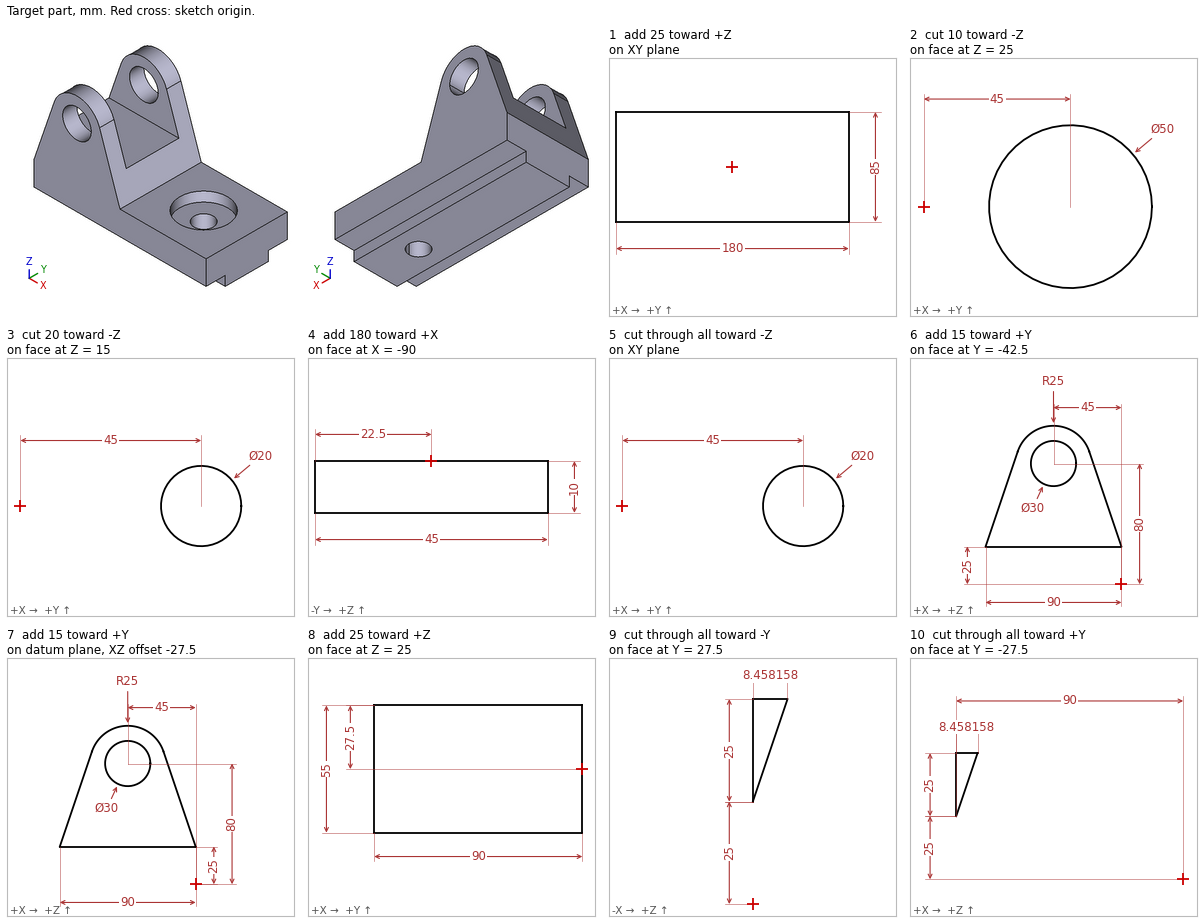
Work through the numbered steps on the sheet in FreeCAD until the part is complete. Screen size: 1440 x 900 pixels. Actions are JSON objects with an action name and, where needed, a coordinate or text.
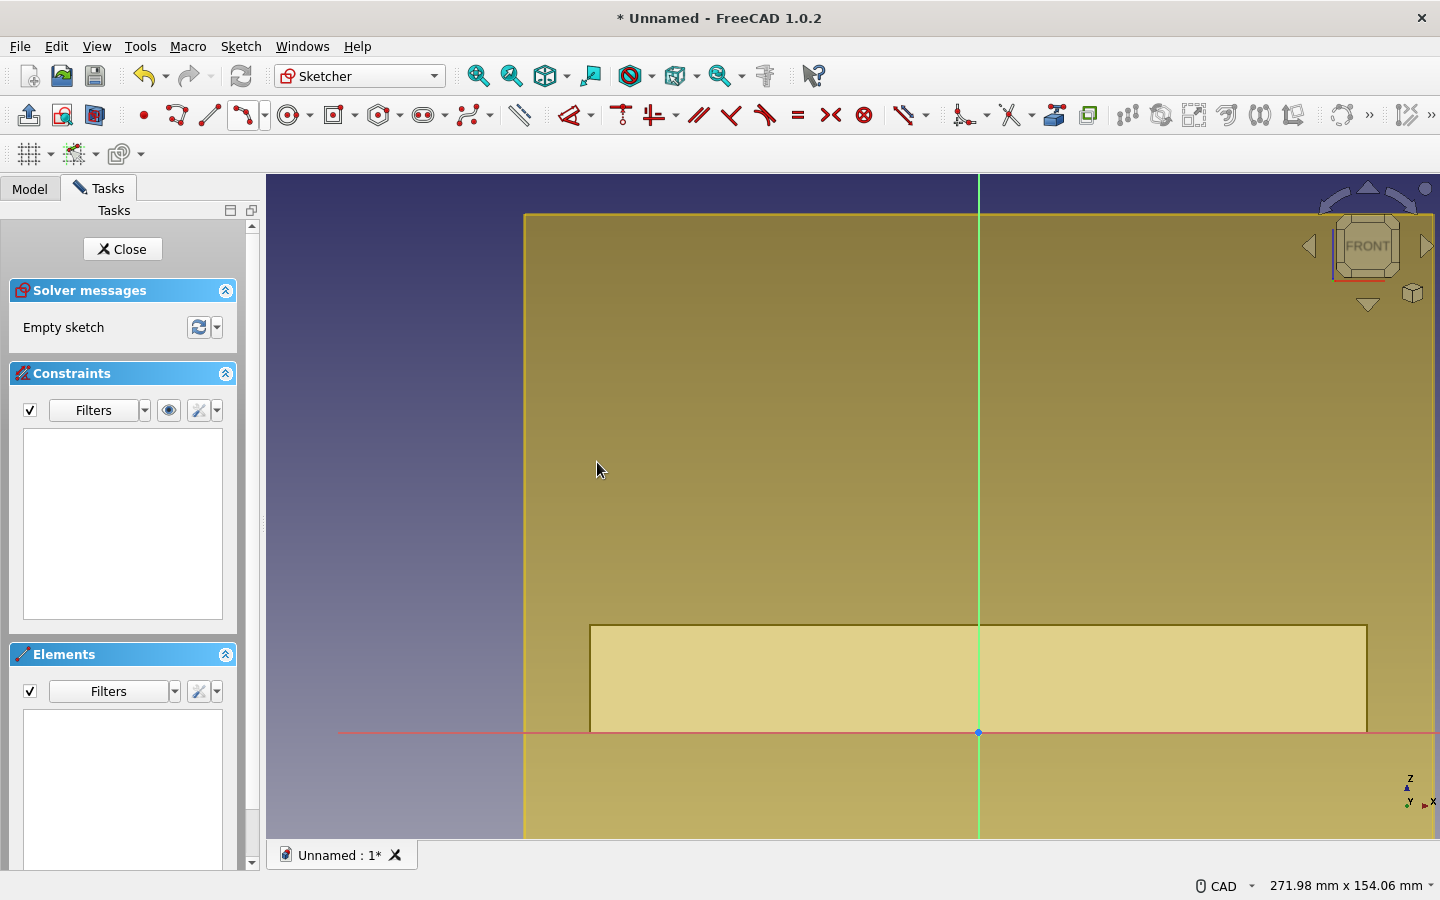
{"action": "left_click", "coordinate": [177, 116]}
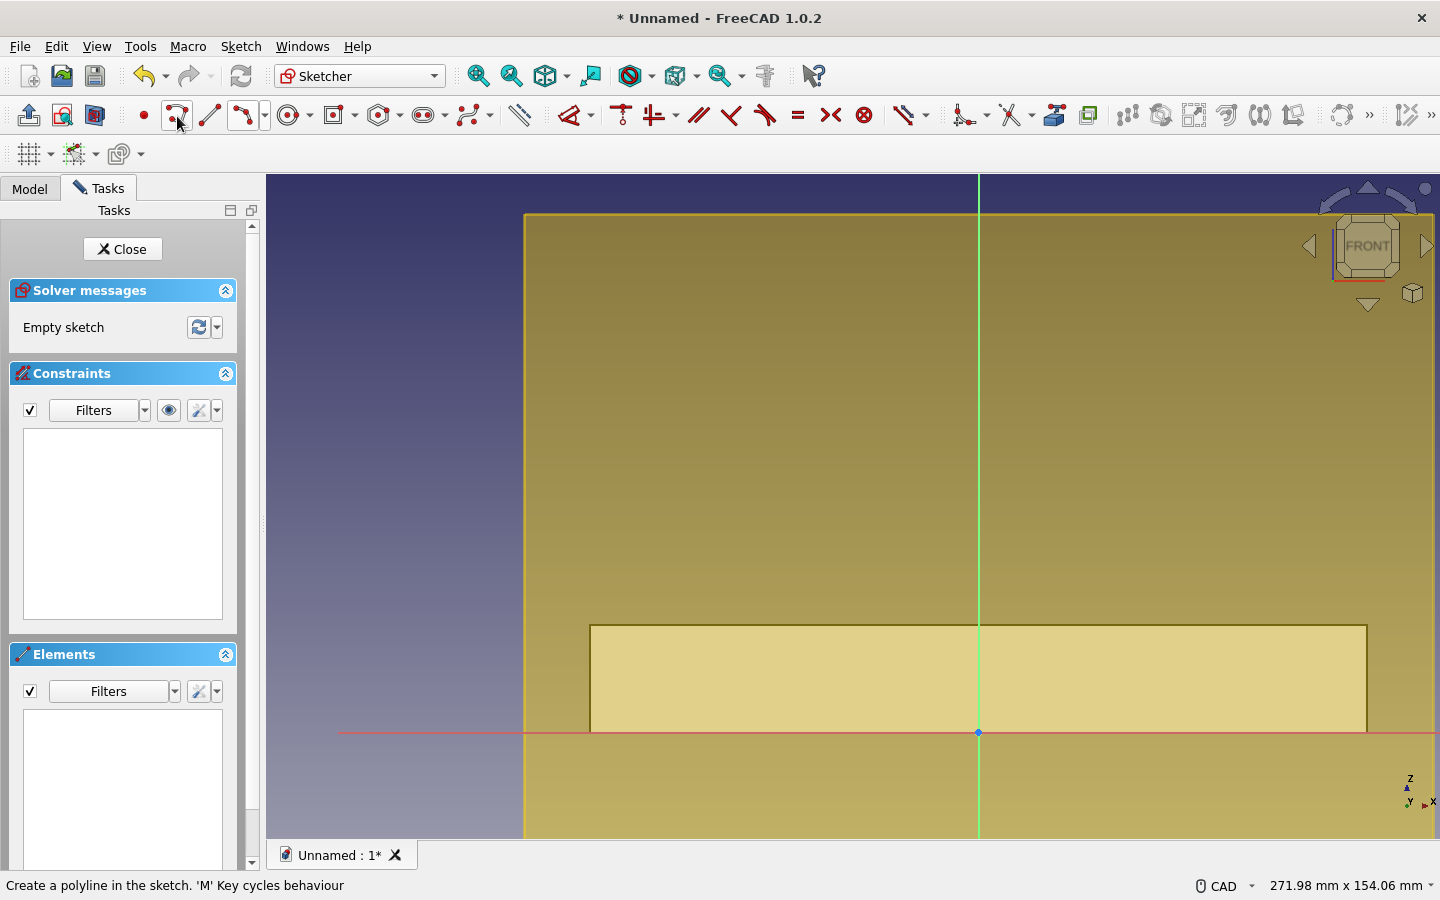
{"action": "left_click", "coordinate": [887, 353]}
{"action": "left_click", "coordinate": [979, 625]}
{"action": "left_click", "coordinate": [590, 625]}
{"action": "left_click", "coordinate": [682, 353]}
{"action": "right_click", "coordinate": [682, 353]}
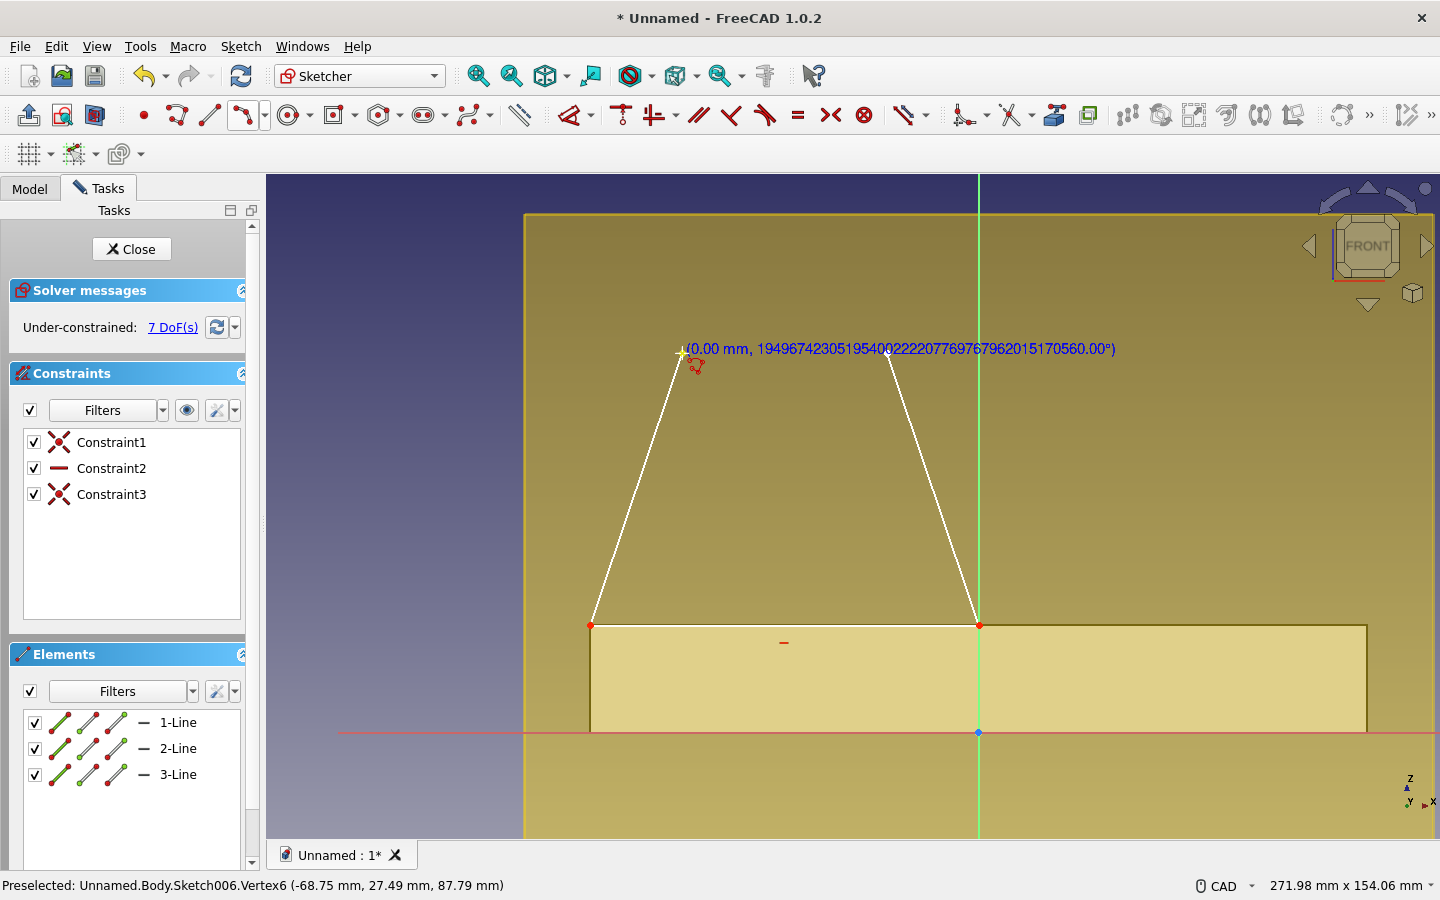
{"action": "left_click", "coordinate": [242, 116]}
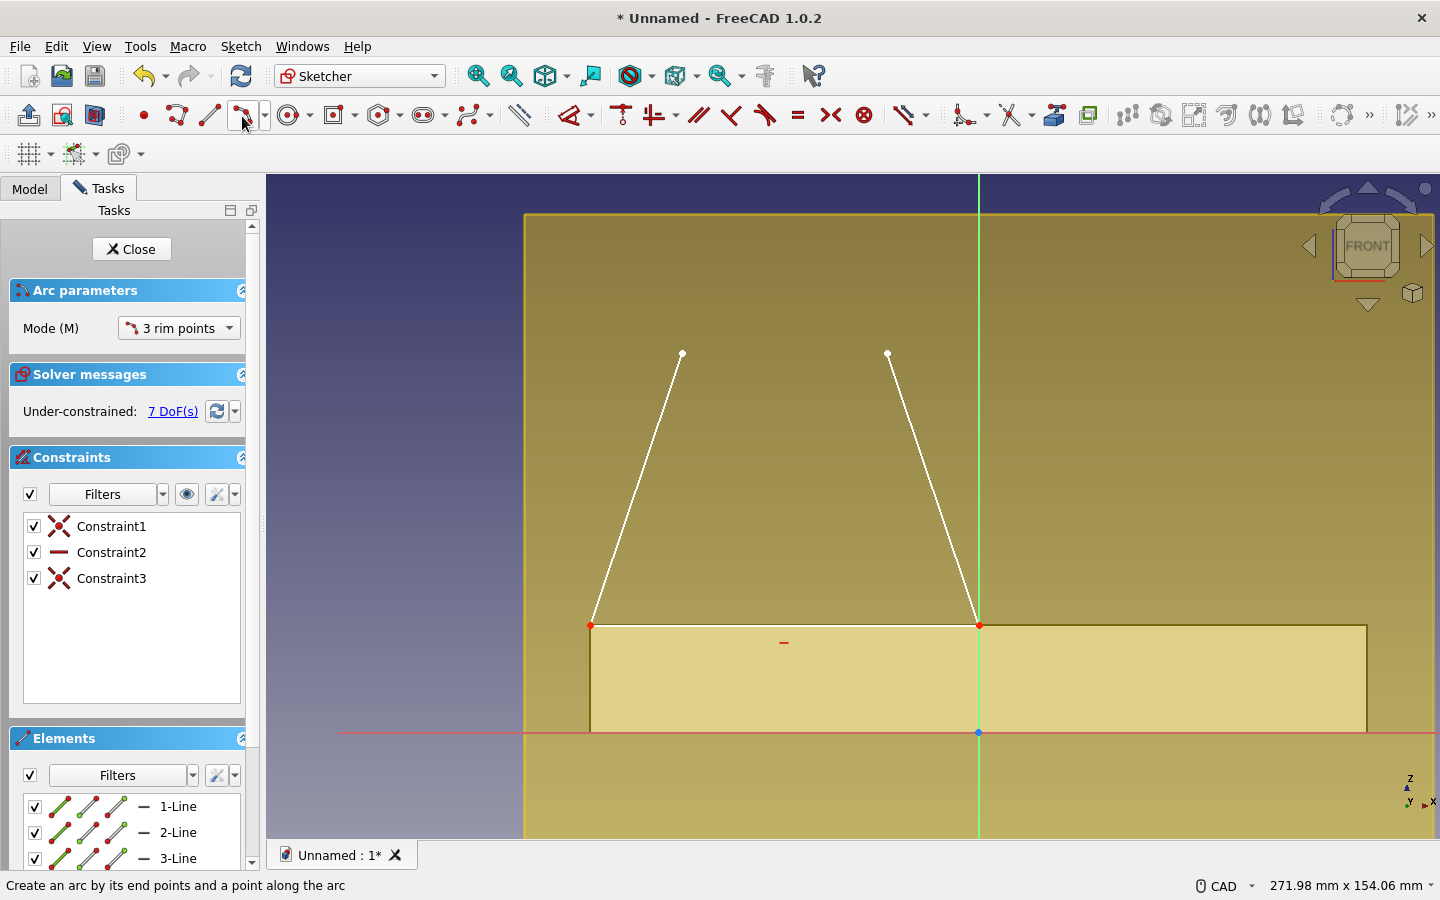
{"action": "left_click", "coordinate": [682, 354]}
{"action": "left_click", "coordinate": [887, 354]}
{"action": "left_click", "coordinate": [785, 280]}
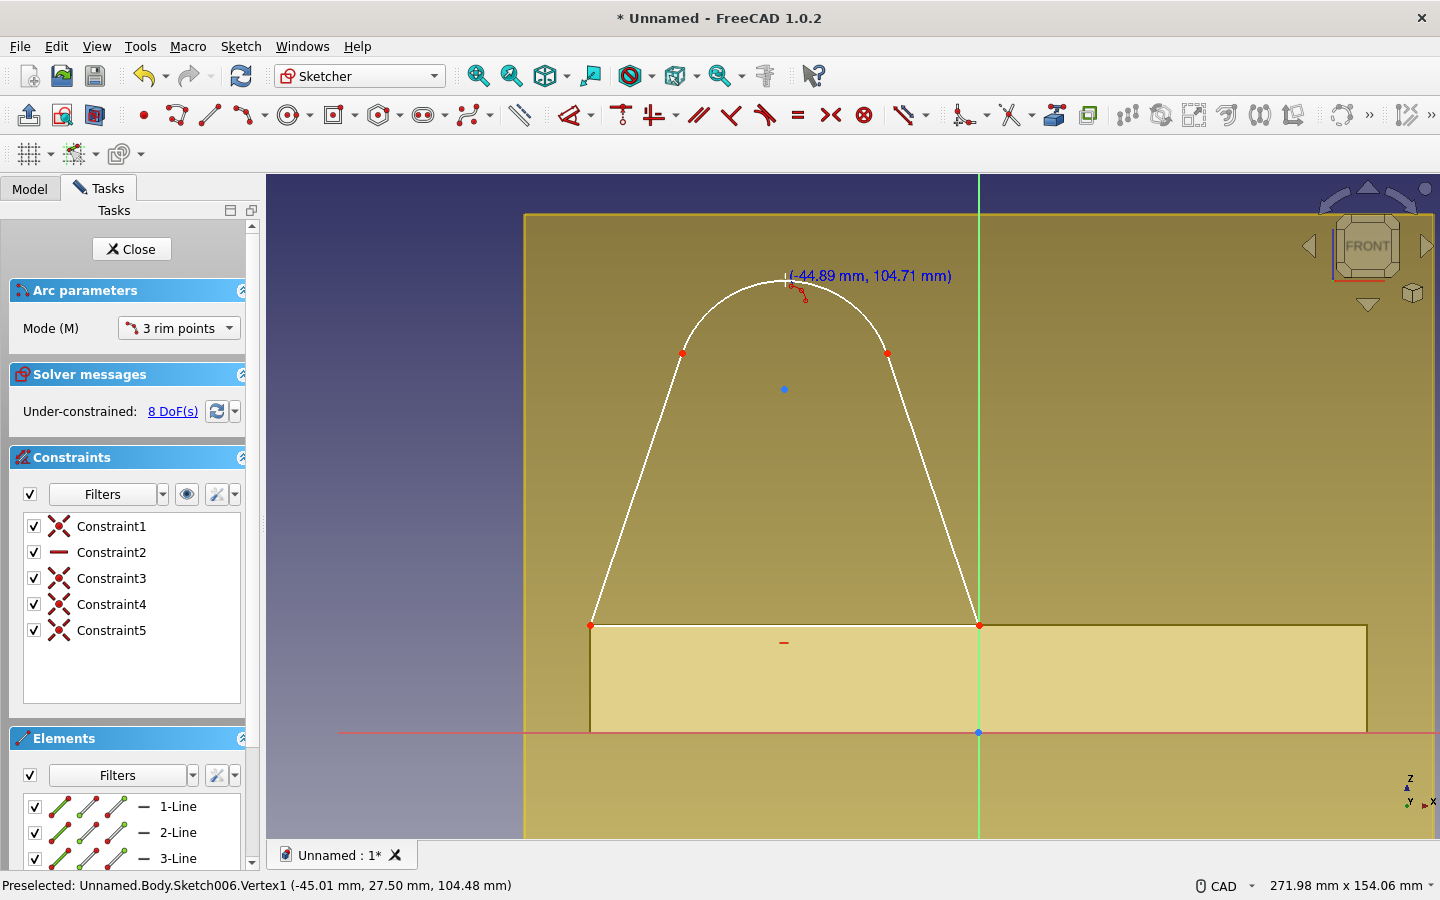
{"action": "left_click", "coordinate": [288, 116]}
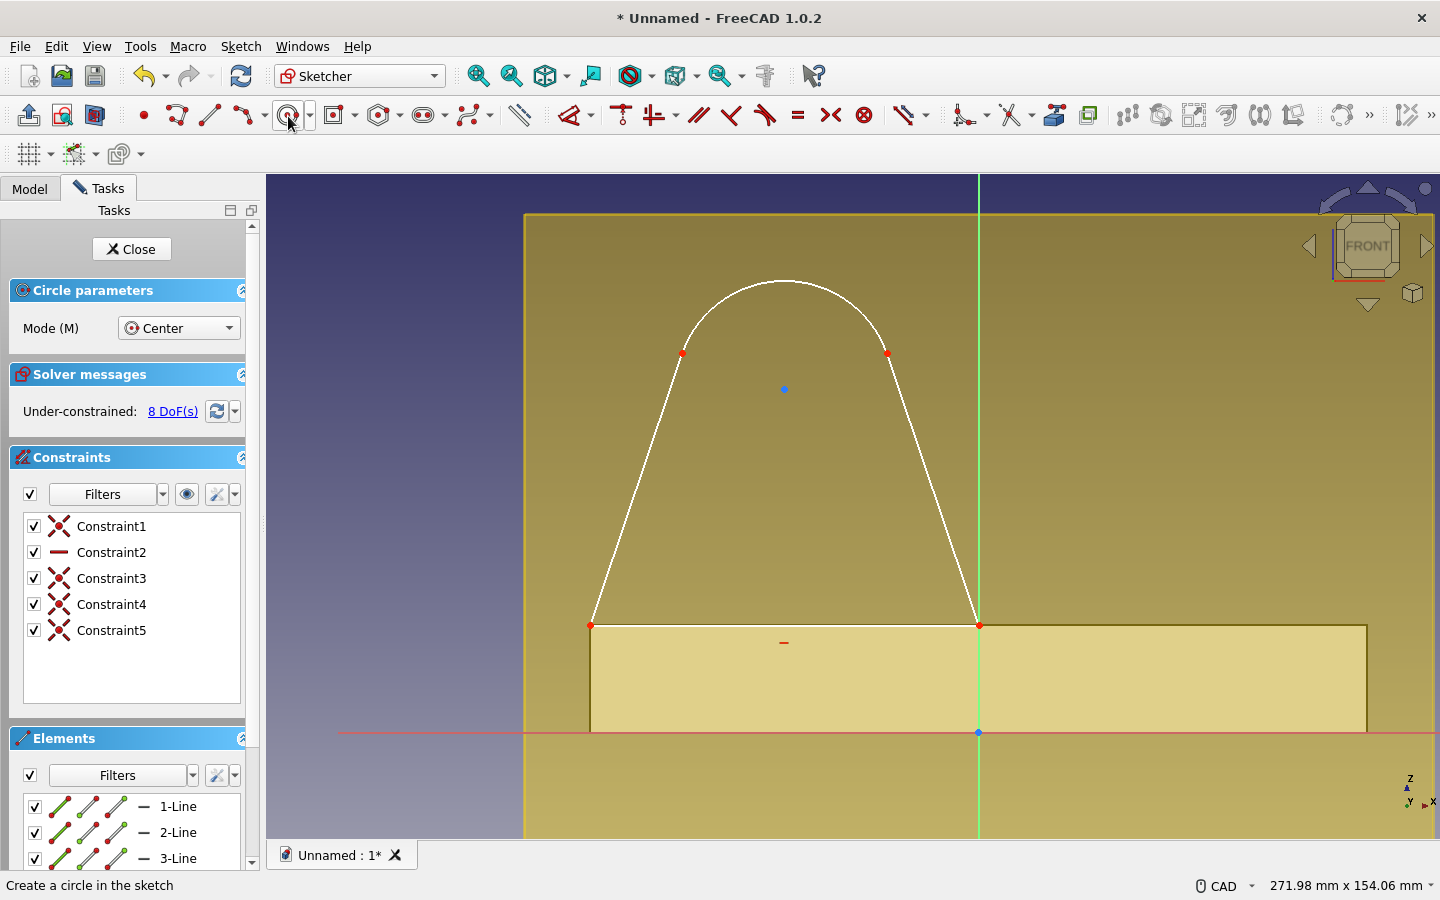
{"action": "left_click", "coordinate": [785, 388]}
{"action": "mouse_move", "coordinate": [830, 342]}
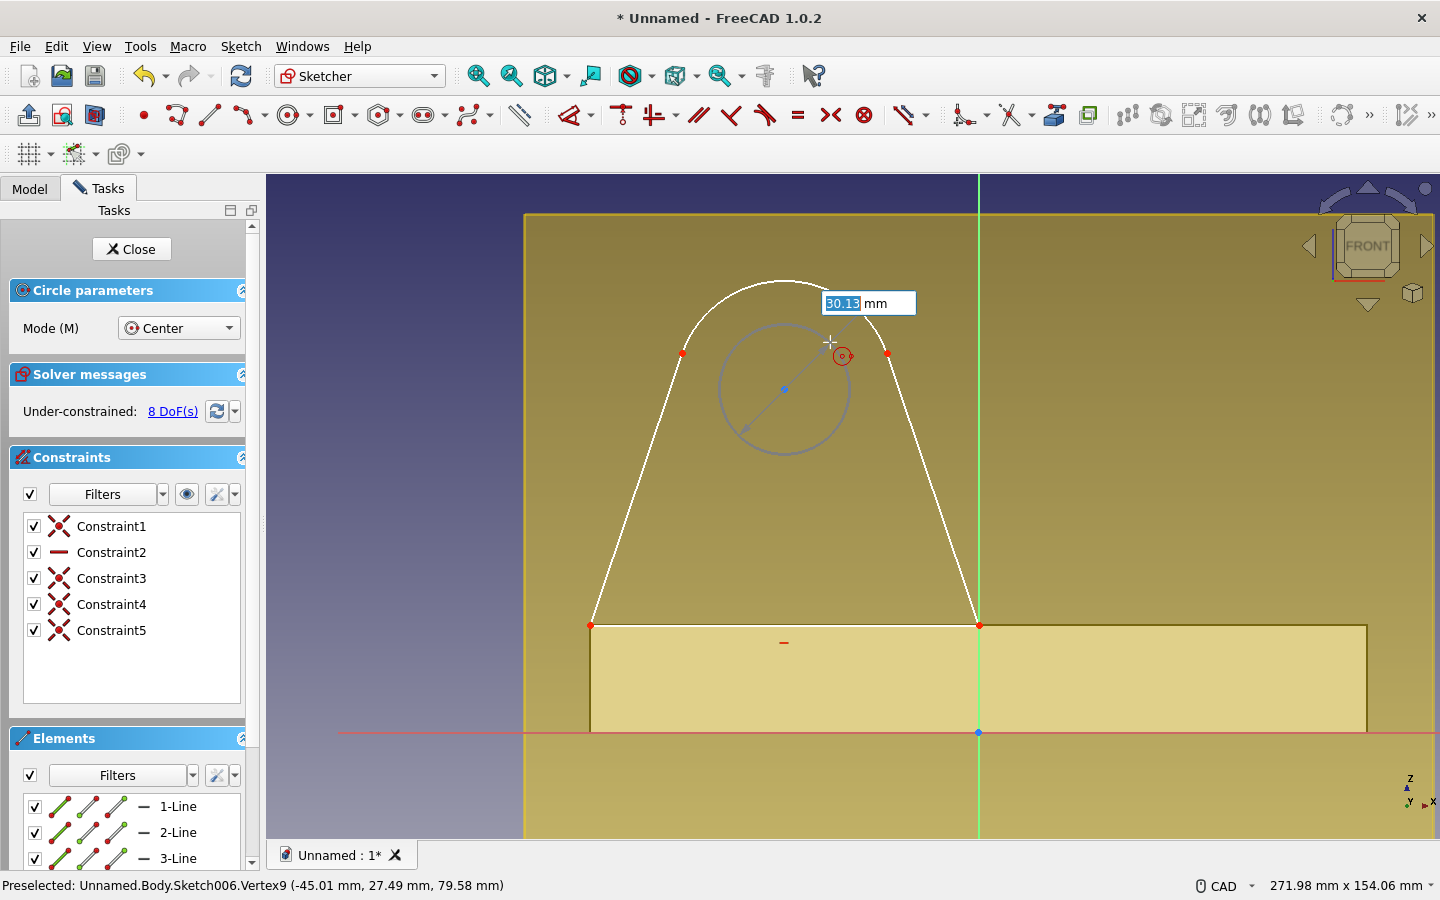
{"action": "type", "text": "30"}
{"action": "key", "text": "Return"}
{"action": "key", "text": "Escape"}